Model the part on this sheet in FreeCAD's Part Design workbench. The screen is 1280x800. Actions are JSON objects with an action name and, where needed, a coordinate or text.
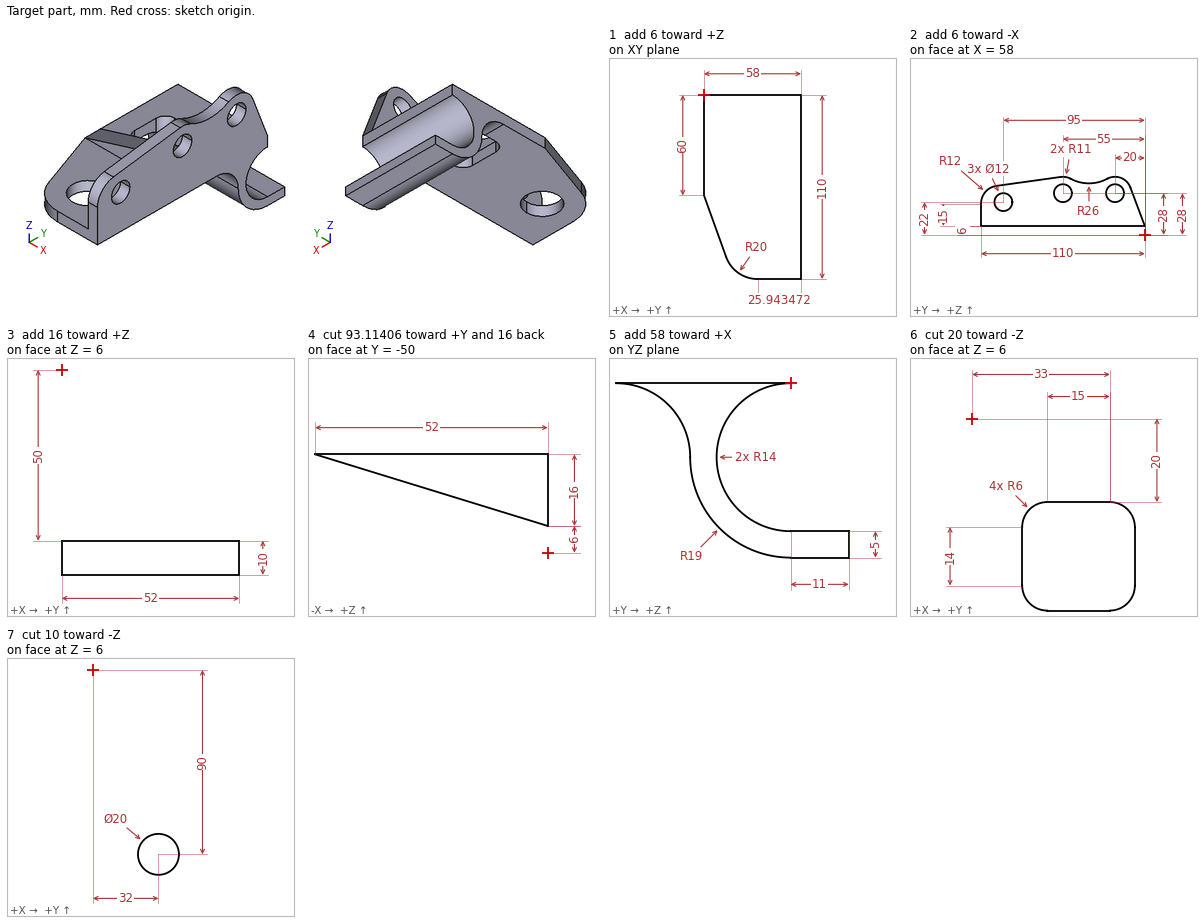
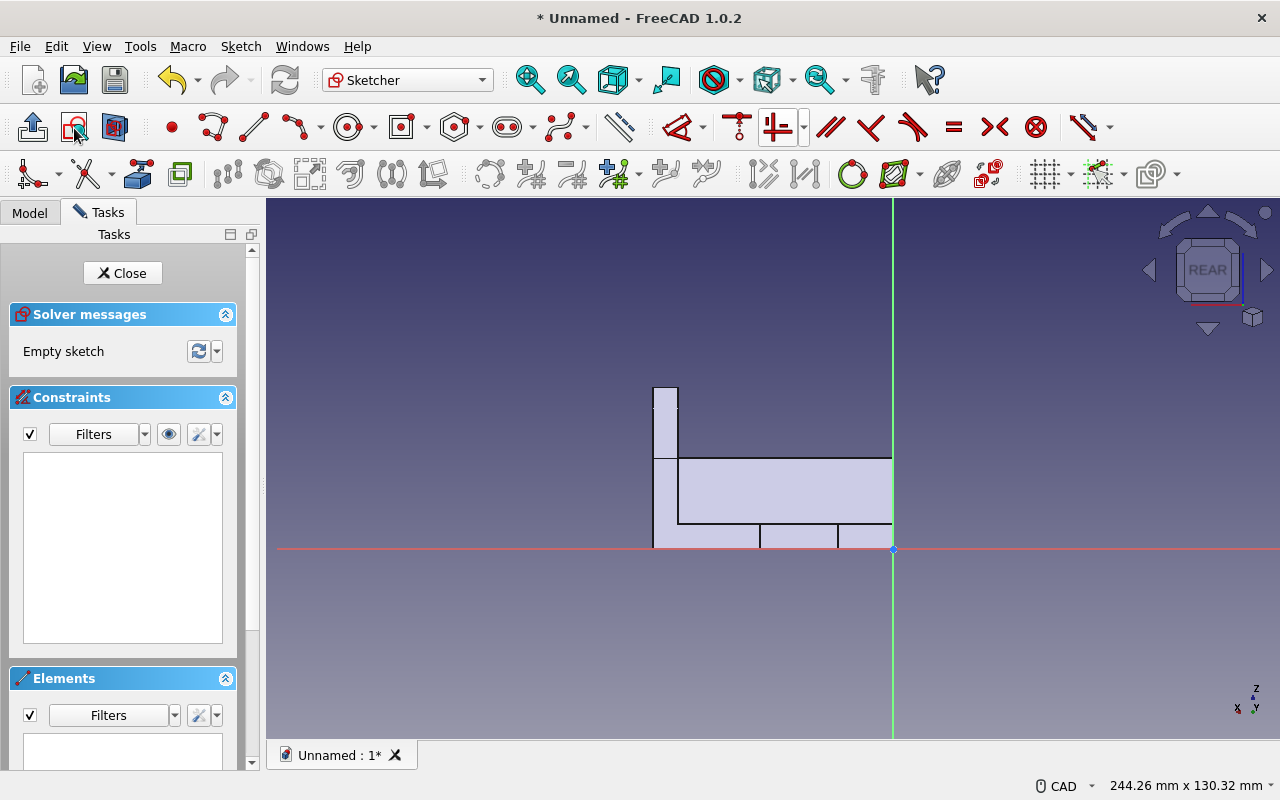
{"action": "scroll", "coordinate": [833, 524], "scroll_direction": "up", "scroll_amount": 5}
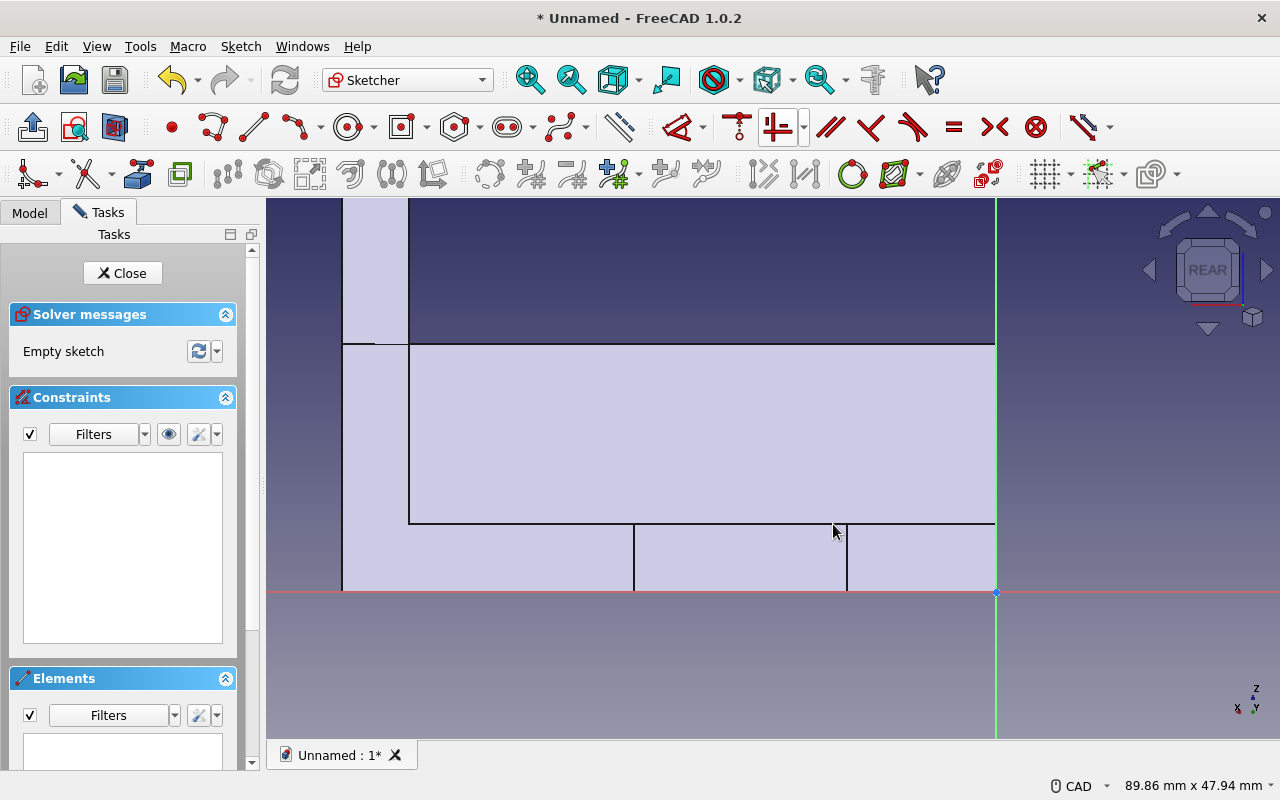
{"action": "left_click", "coordinate": [213, 128]}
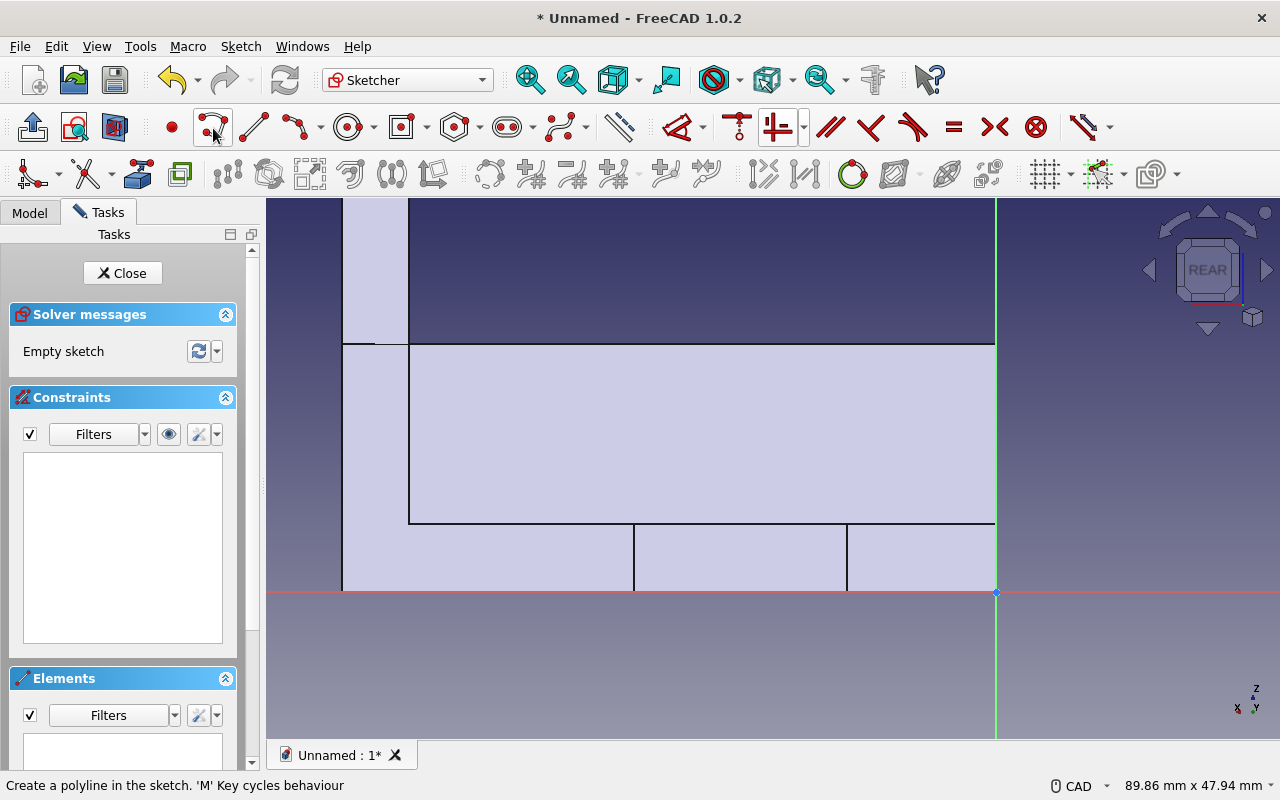
{"action": "left_click", "coordinate": [996, 524]}
{"action": "left_click", "coordinate": [987, 344]}
{"action": "left_click", "coordinate": [409, 344]}
{"action": "left_click", "coordinate": [996, 525]}
{"action": "key", "text": "Escape"}
{"action": "key", "text": "Escape"}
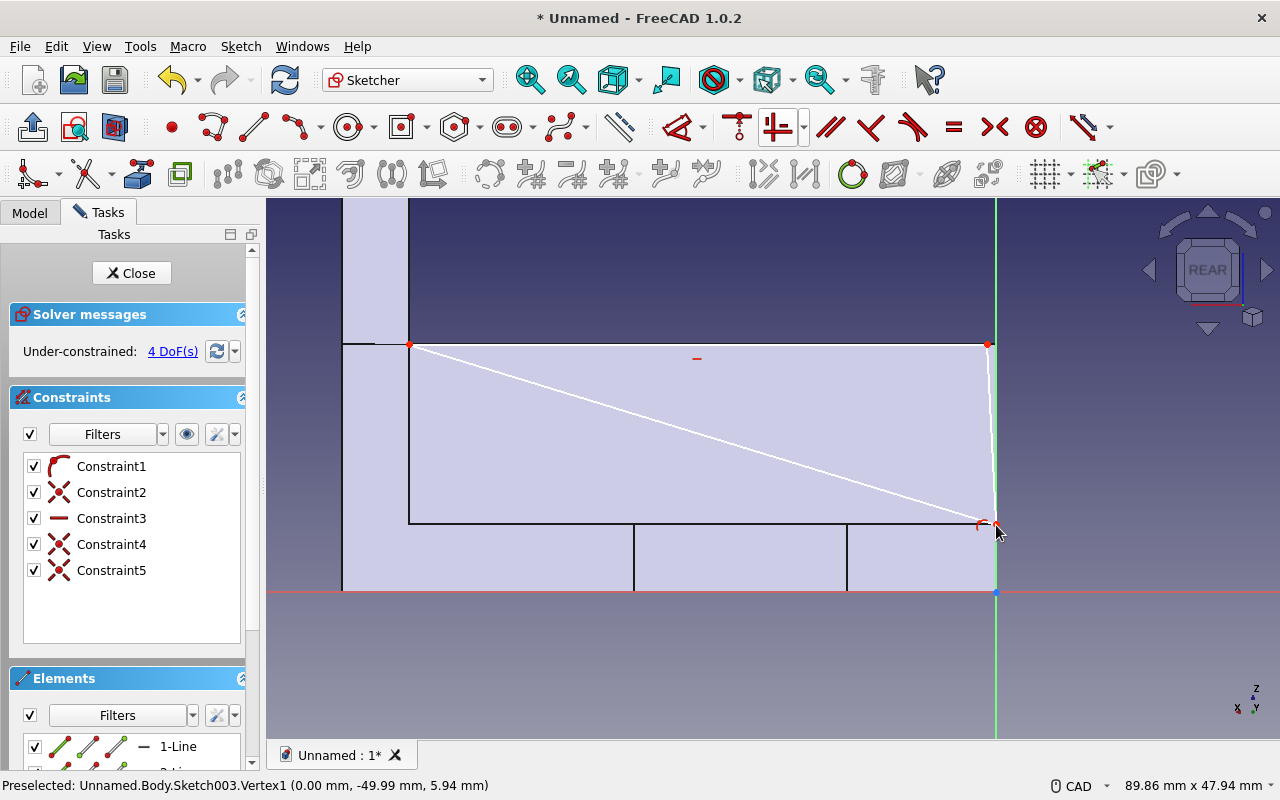
{"action": "left_click", "coordinate": [993, 471]}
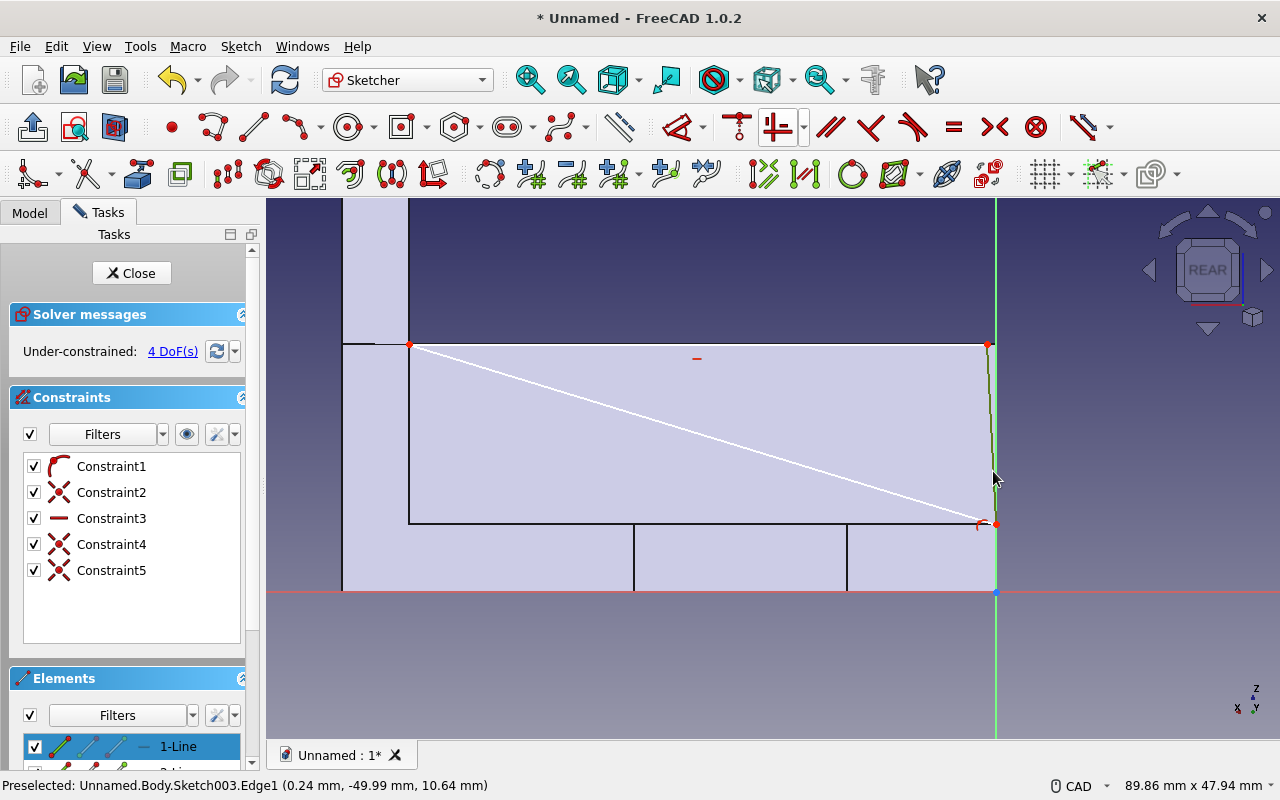
{"action": "key", "text": "v"}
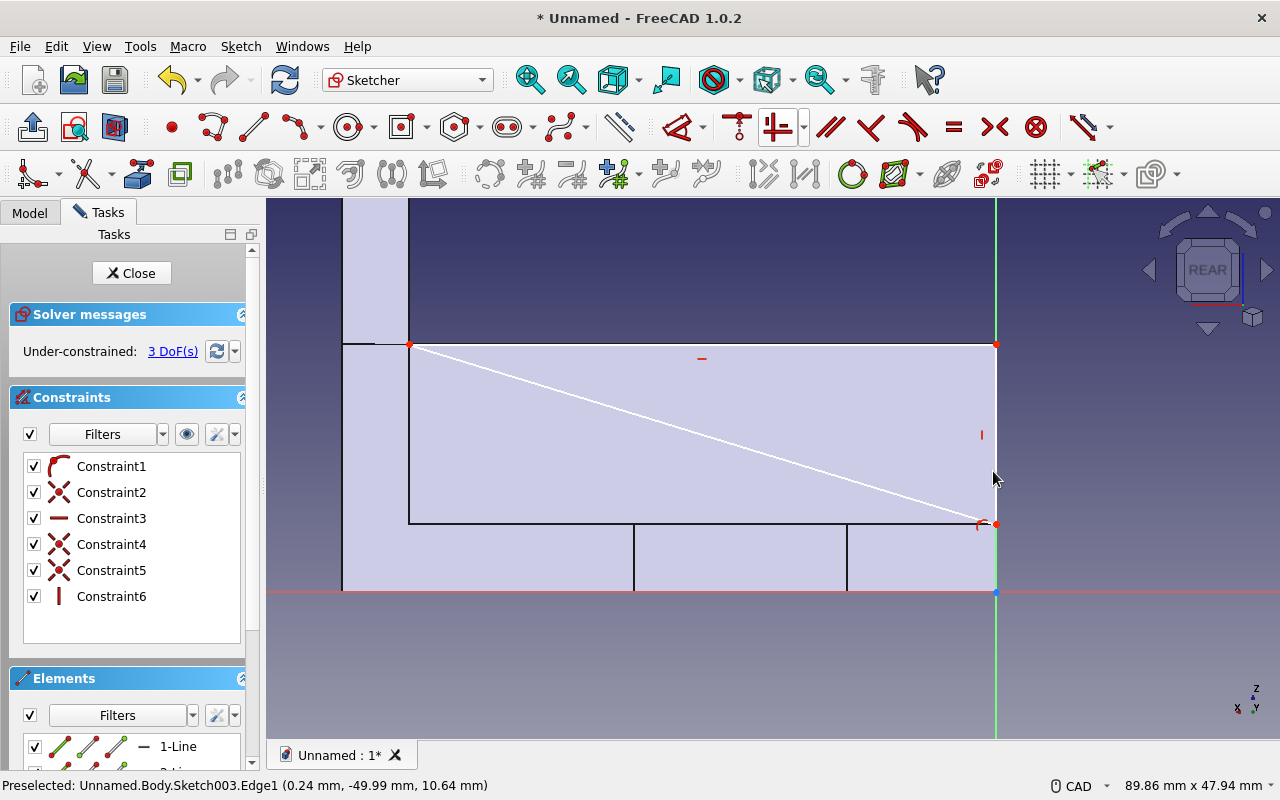
{"action": "left_click", "coordinate": [676, 128]}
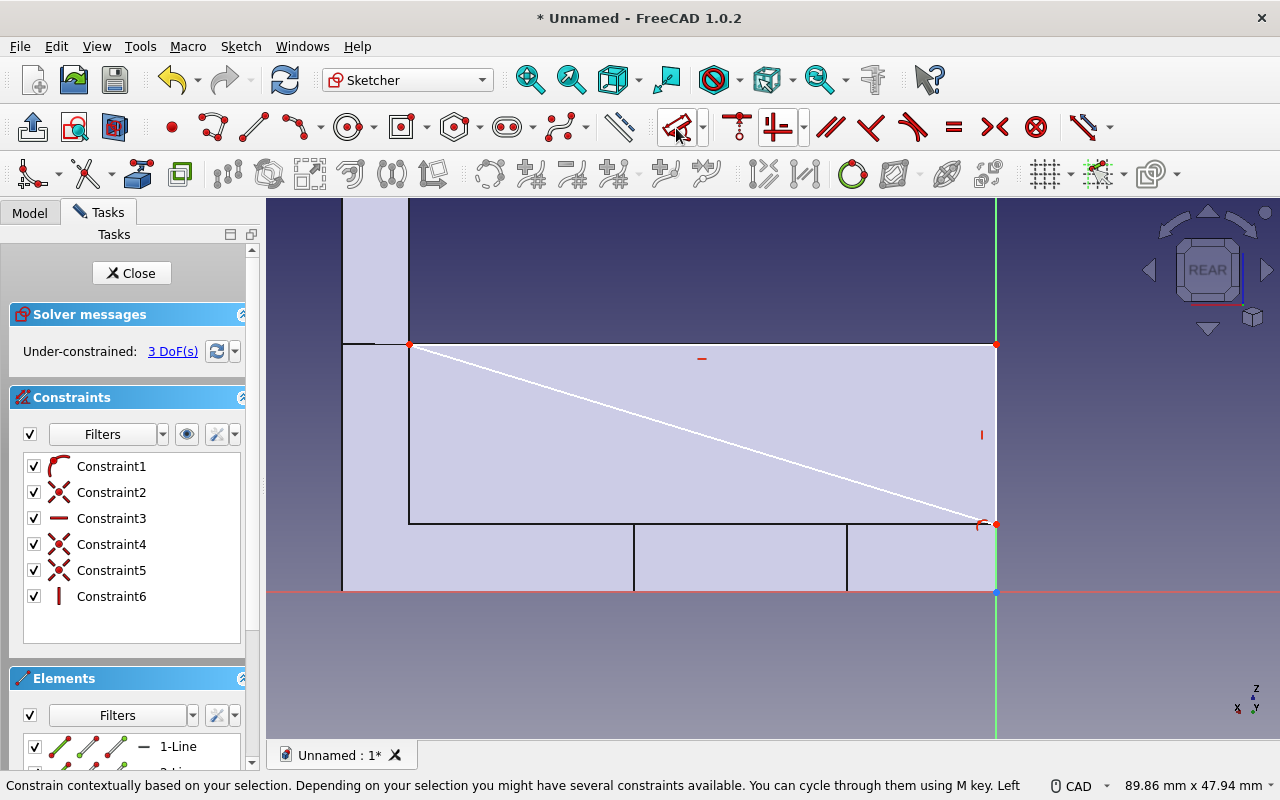
{"action": "left_click", "coordinate": [996, 471]}
{"action": "left_click", "coordinate": [1030, 435]}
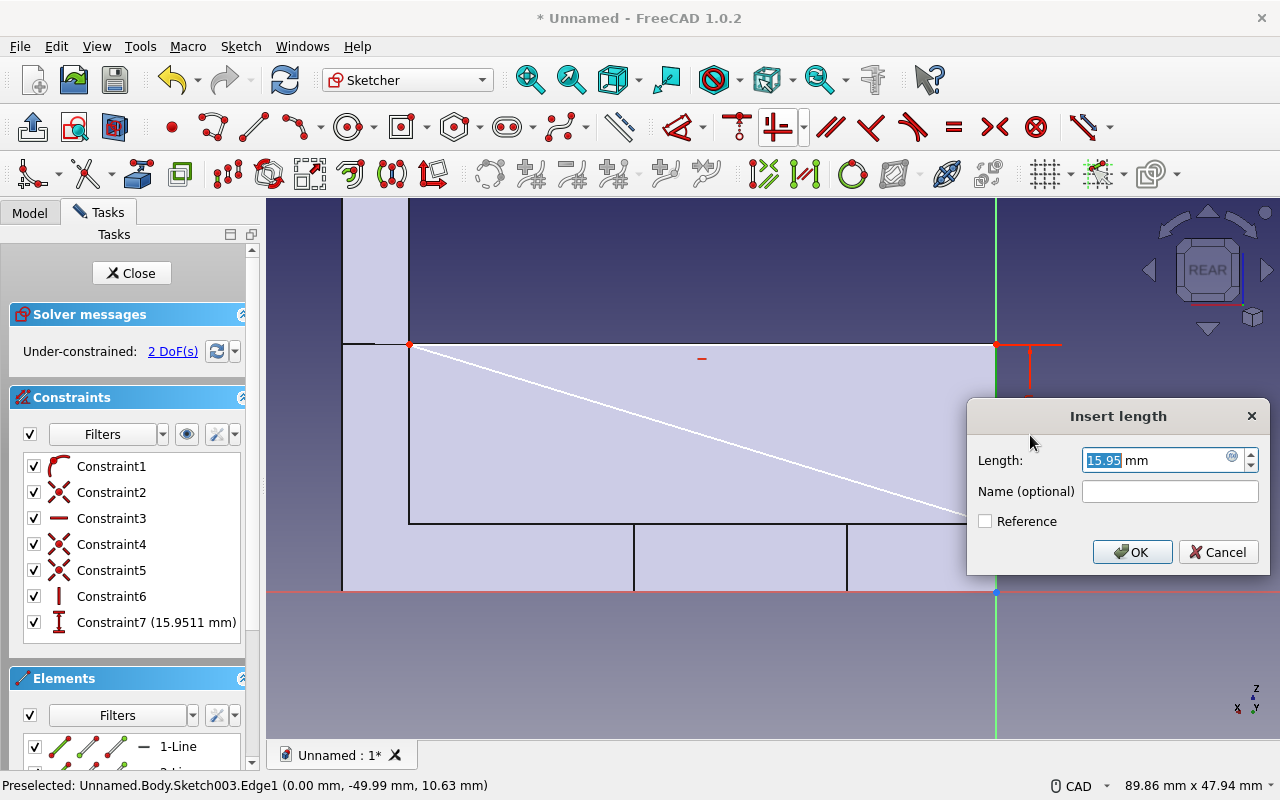
{"action": "type", "text": "16"}
{"action": "key", "text": "Return"}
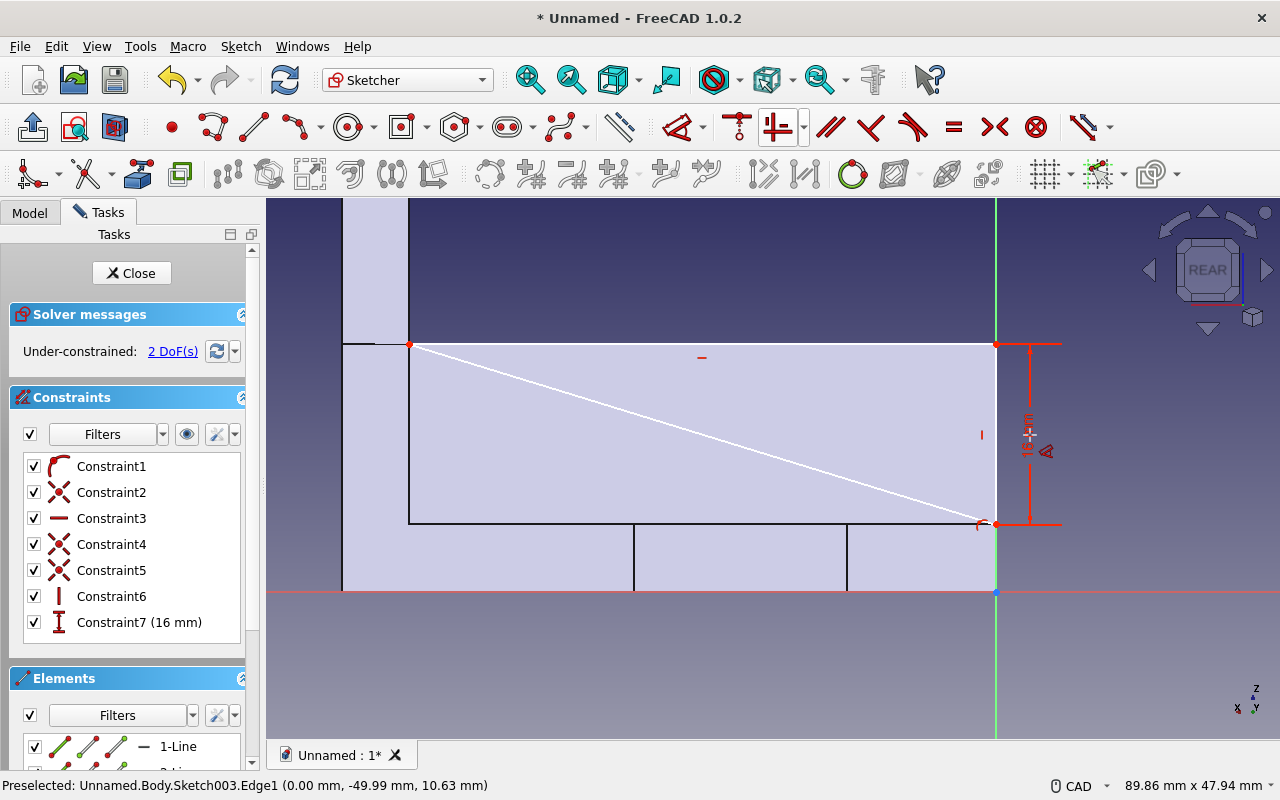
{"action": "left_click", "coordinate": [820, 344]}
{"action": "left_click", "coordinate": [703, 310]}